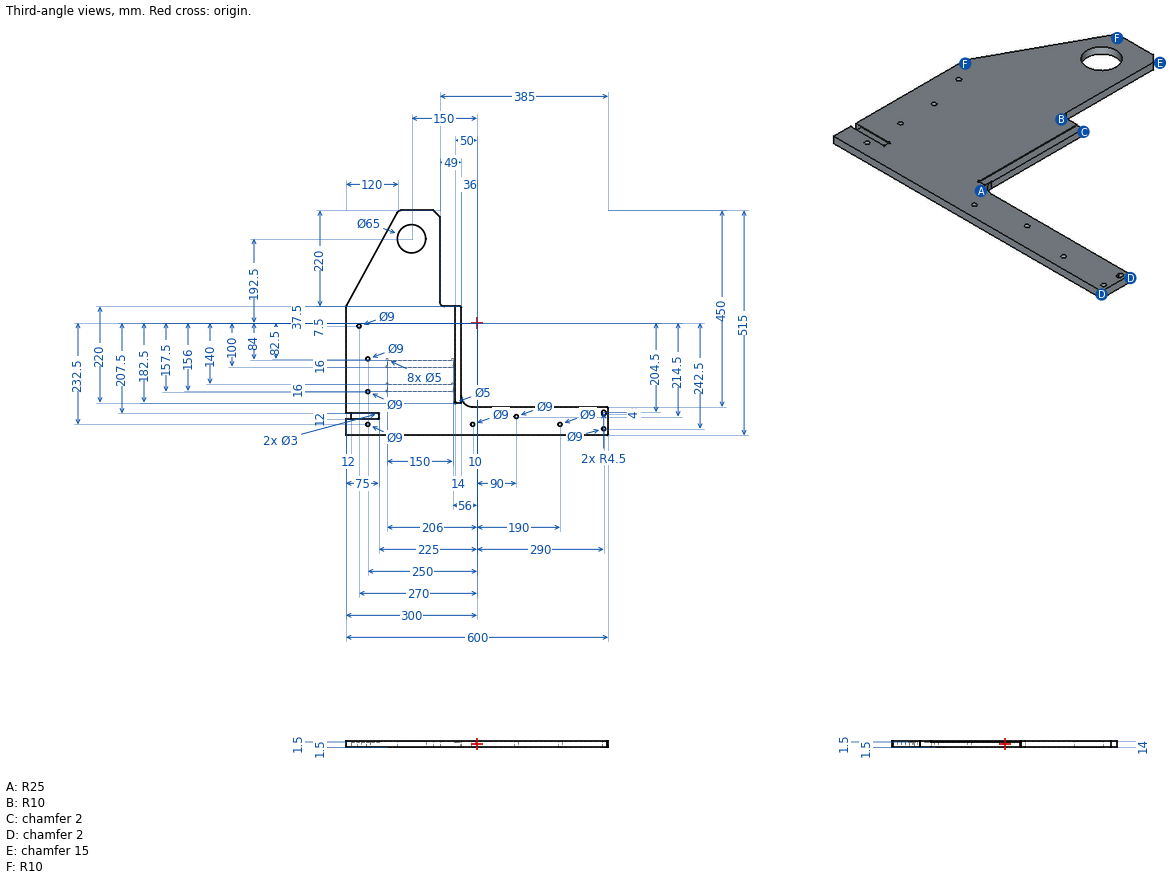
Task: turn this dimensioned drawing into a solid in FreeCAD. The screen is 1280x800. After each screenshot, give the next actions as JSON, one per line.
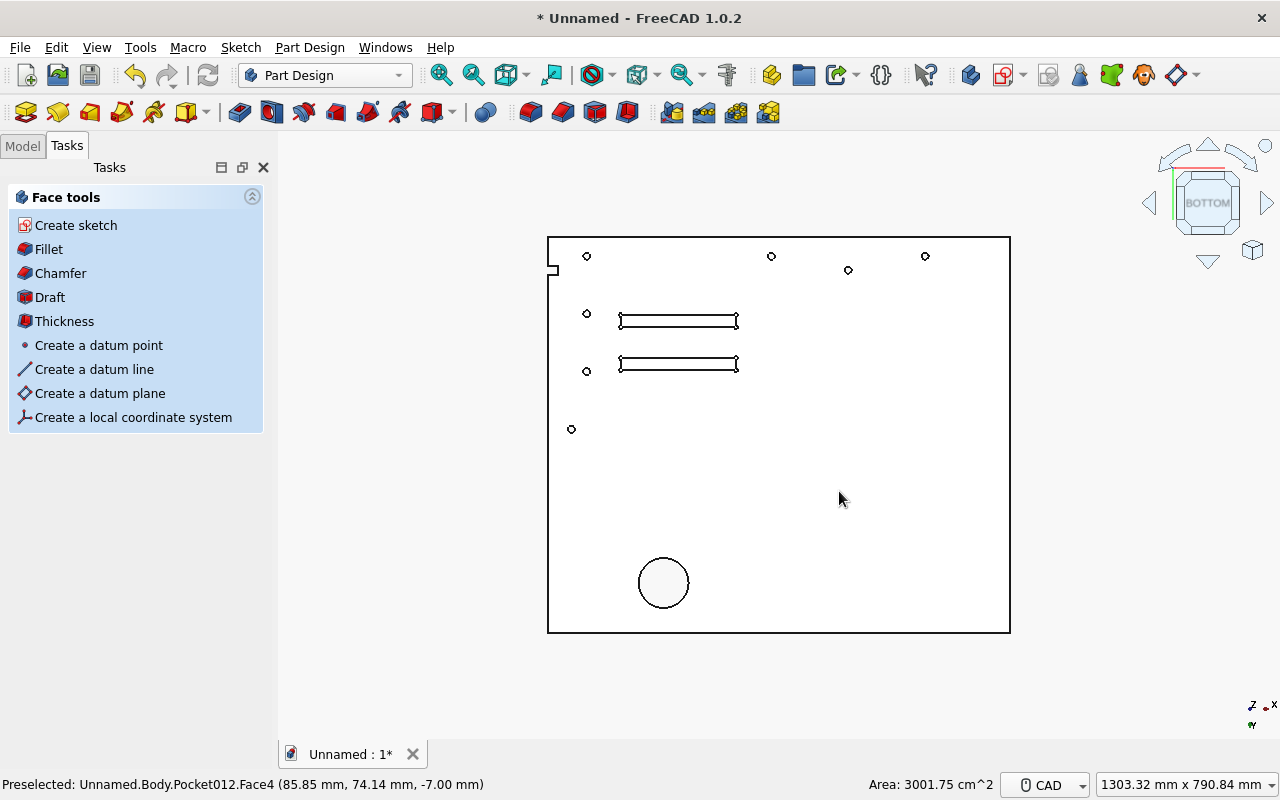
{"action": "left_click", "coordinate": [1004, 76]}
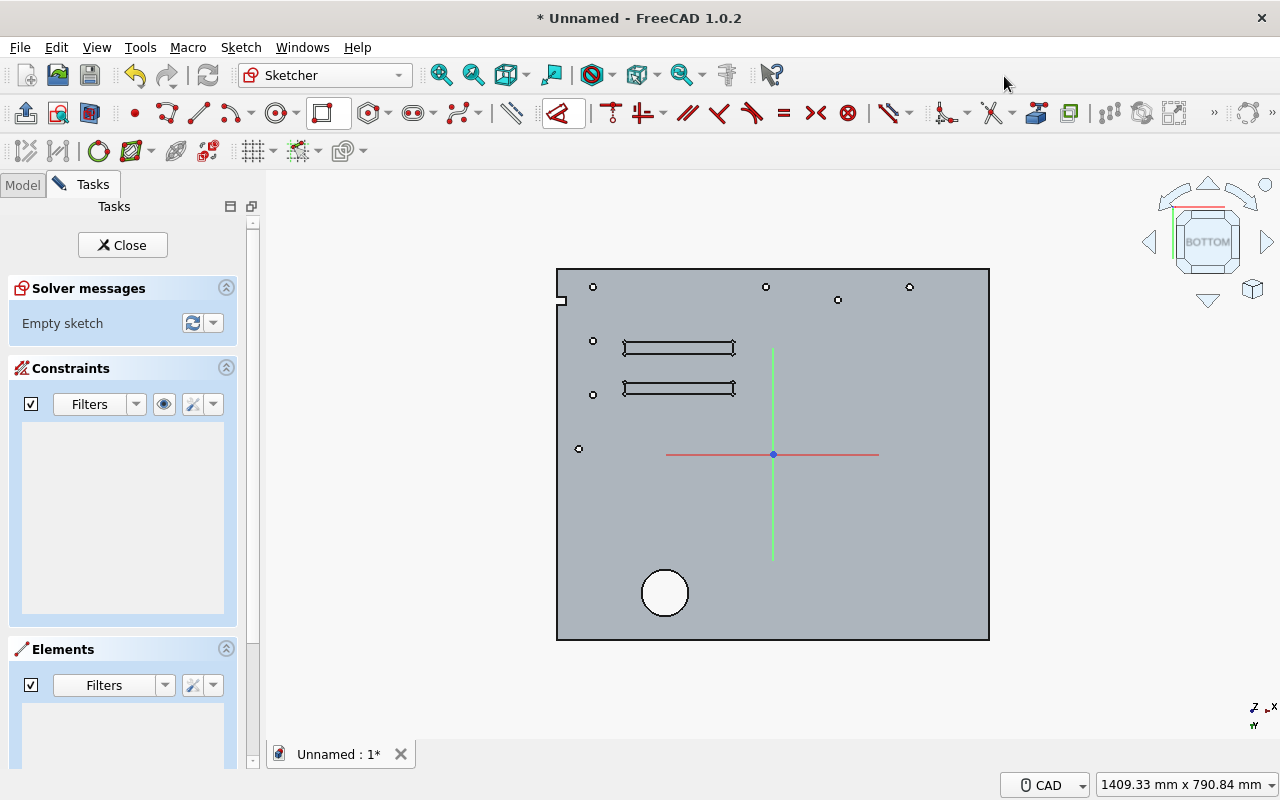
{"action": "scroll", "coordinate": [996, 271], "scroll_direction": "up", "scroll_amount": 15}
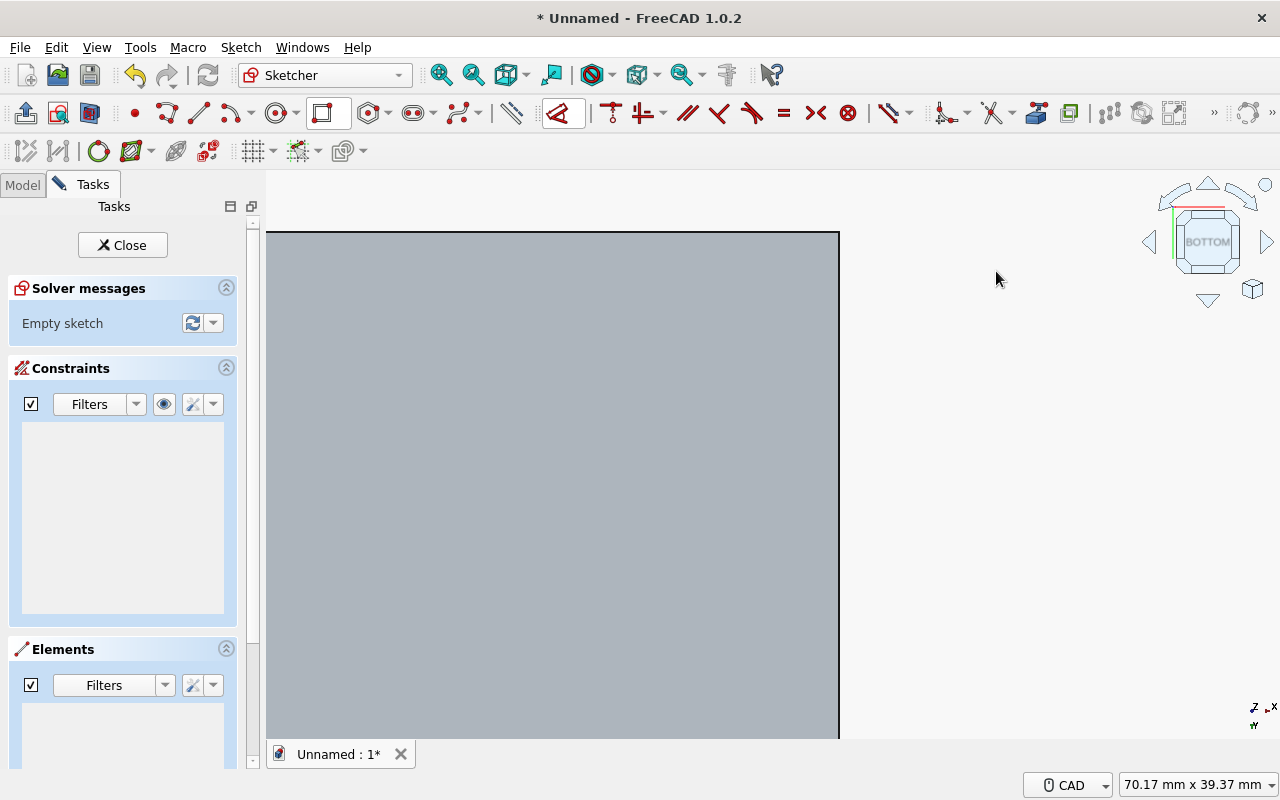
{"action": "scroll", "coordinate": [688, 446], "scroll_direction": "up", "scroll_amount": 5}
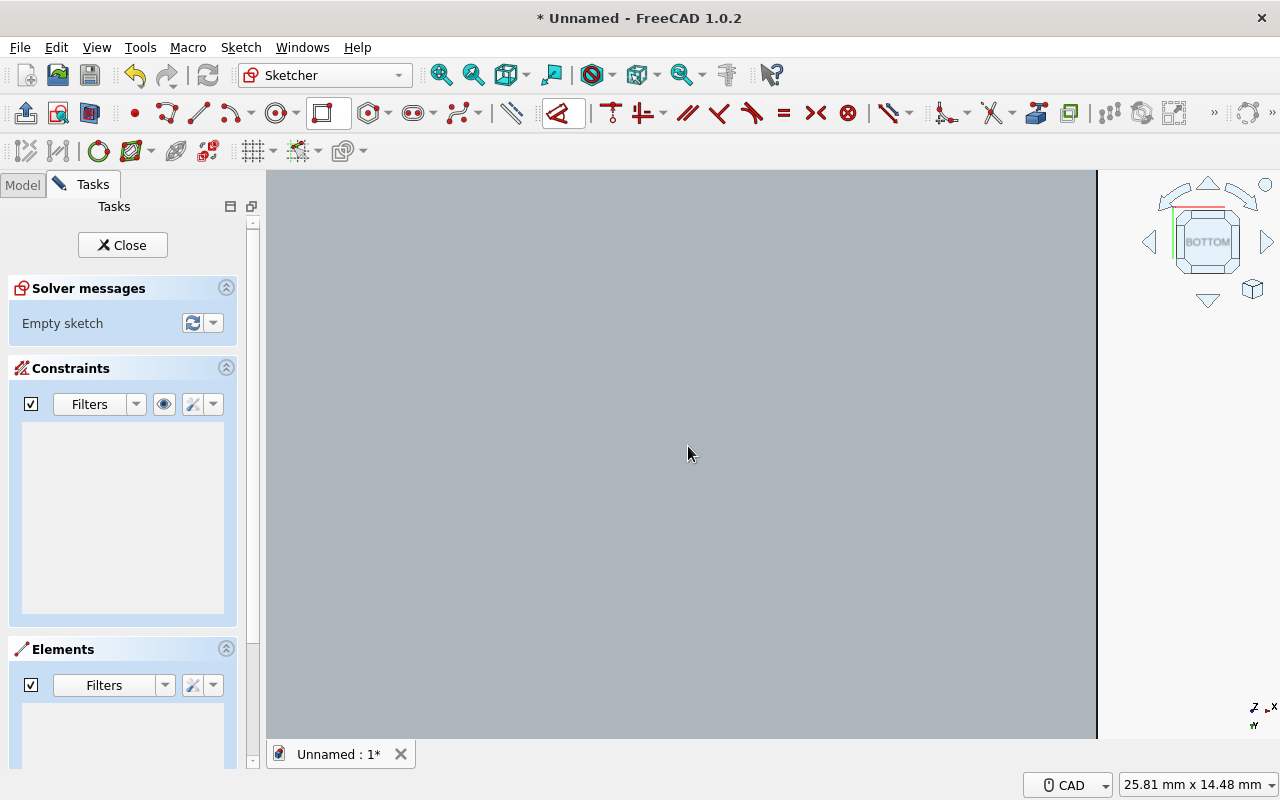
{"action": "left_click", "coordinate": [276, 114]}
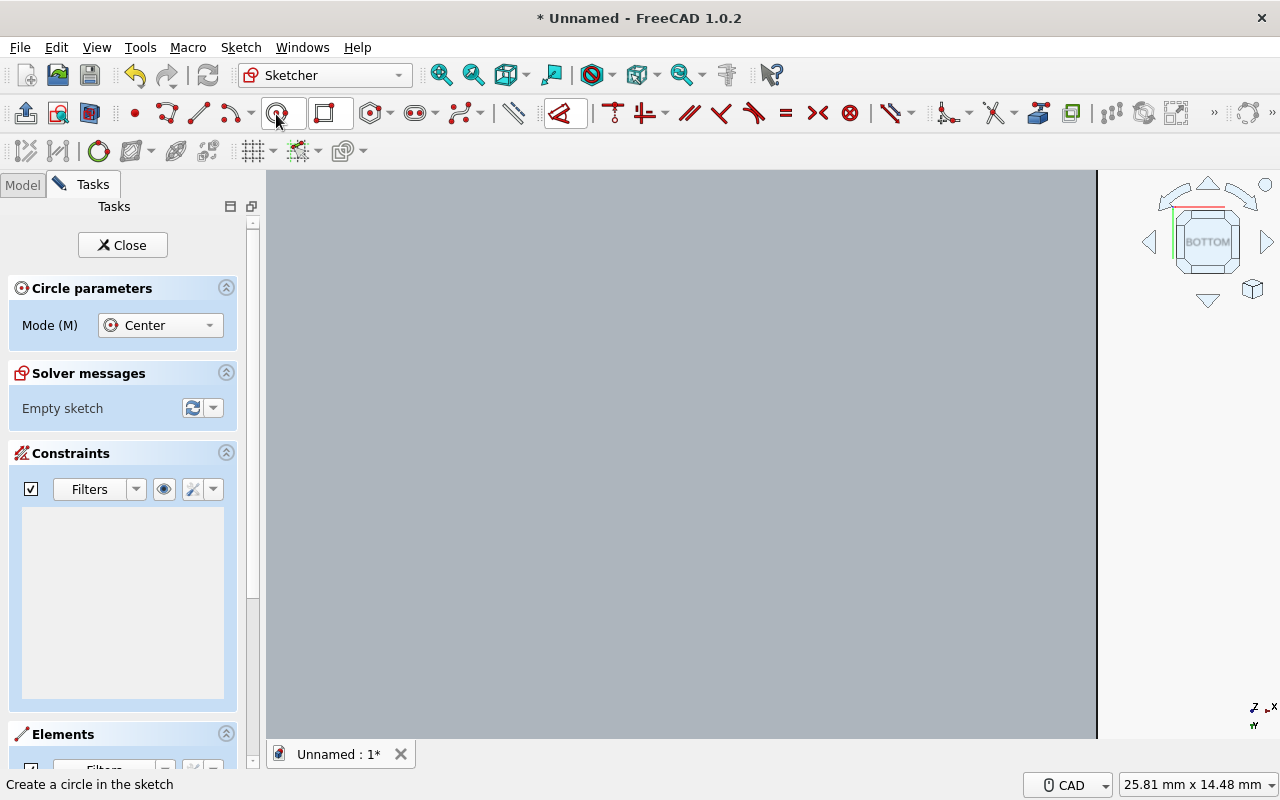
{"action": "left_click", "coordinate": [704, 453]}
{"action": "mouse_move", "coordinate": [829, 328]}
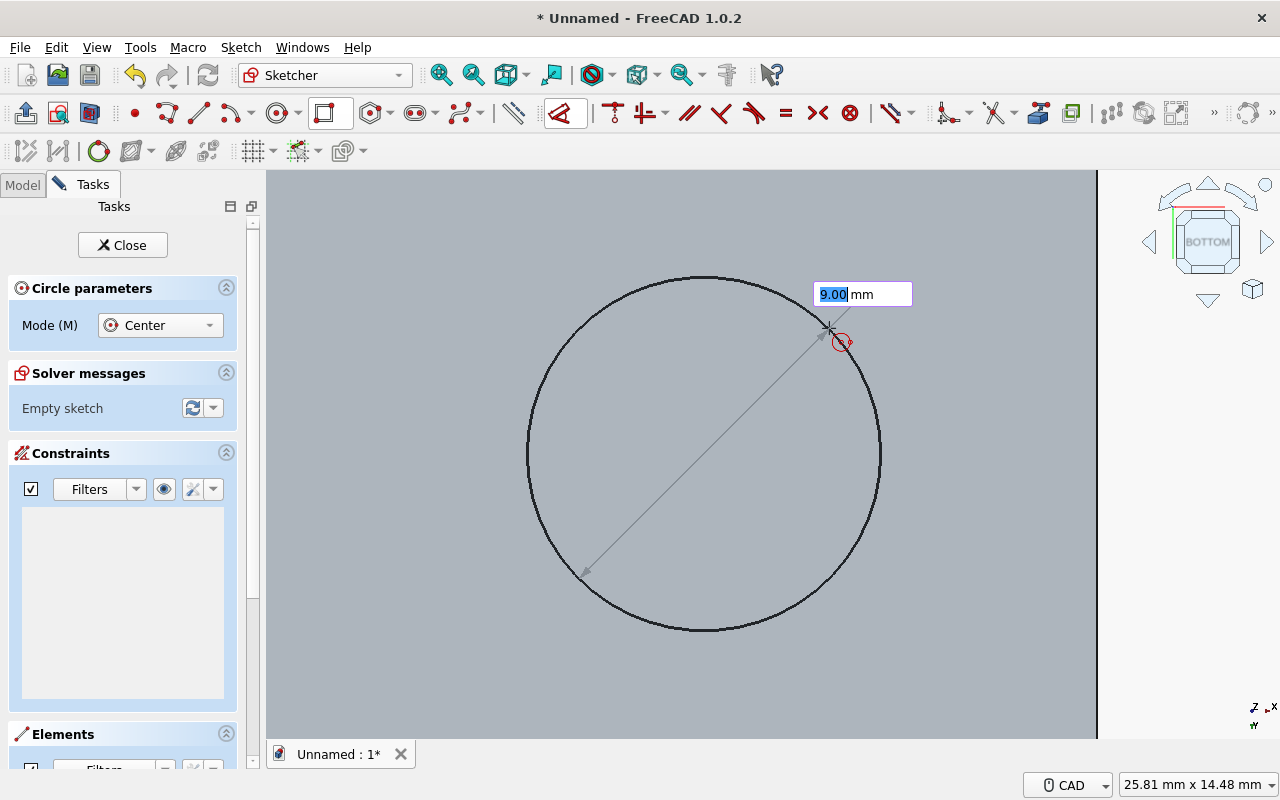
{"action": "type", "text": "9"}
{"action": "key", "text": "Return"}
{"action": "key", "text": "Escape"}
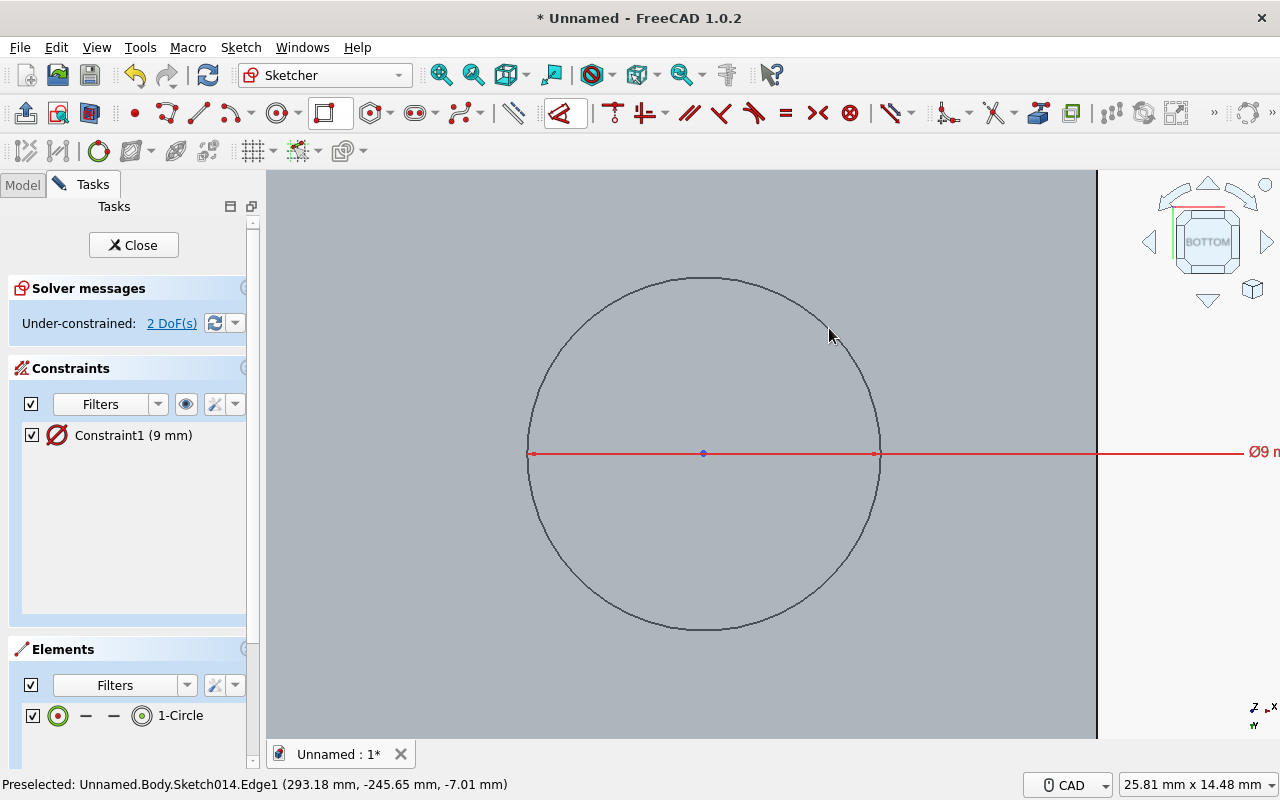
{"action": "left_click", "coordinate": [704, 454]}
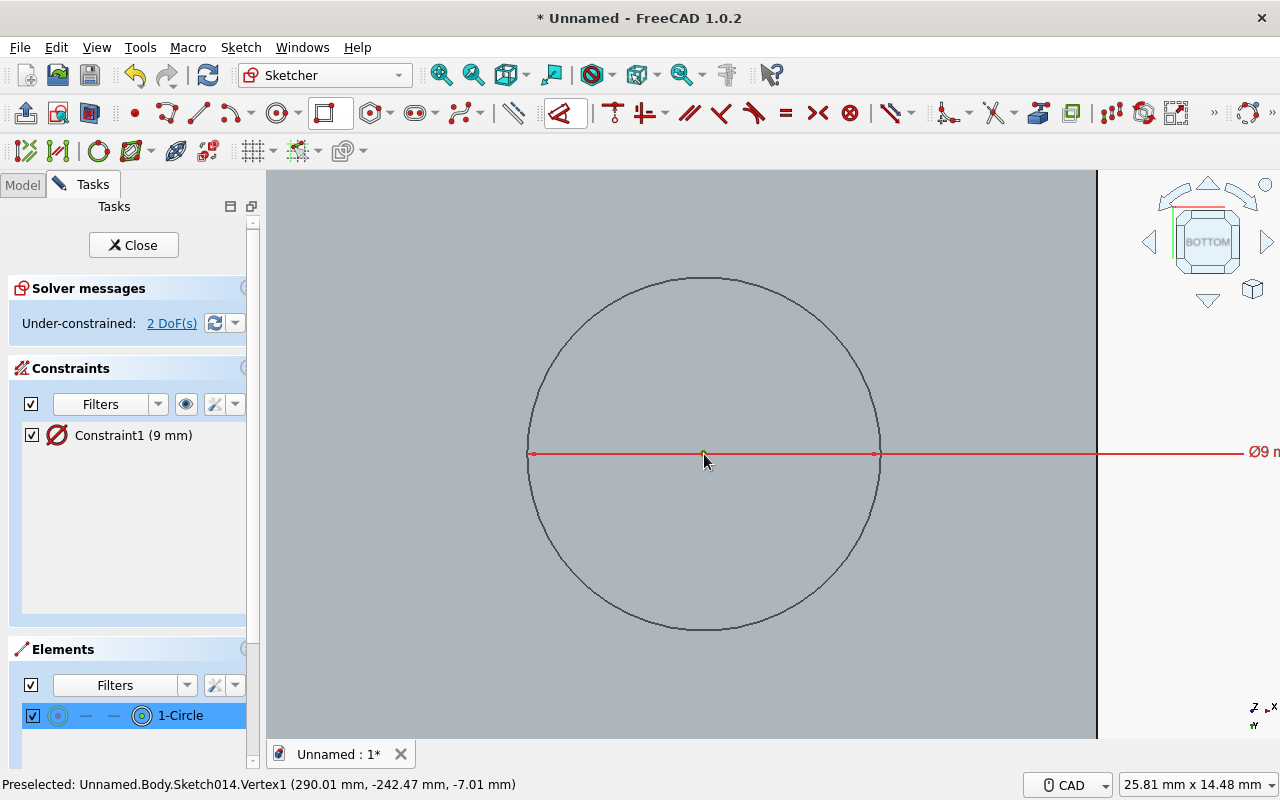
{"action": "left_click", "coordinate": [582, 114]}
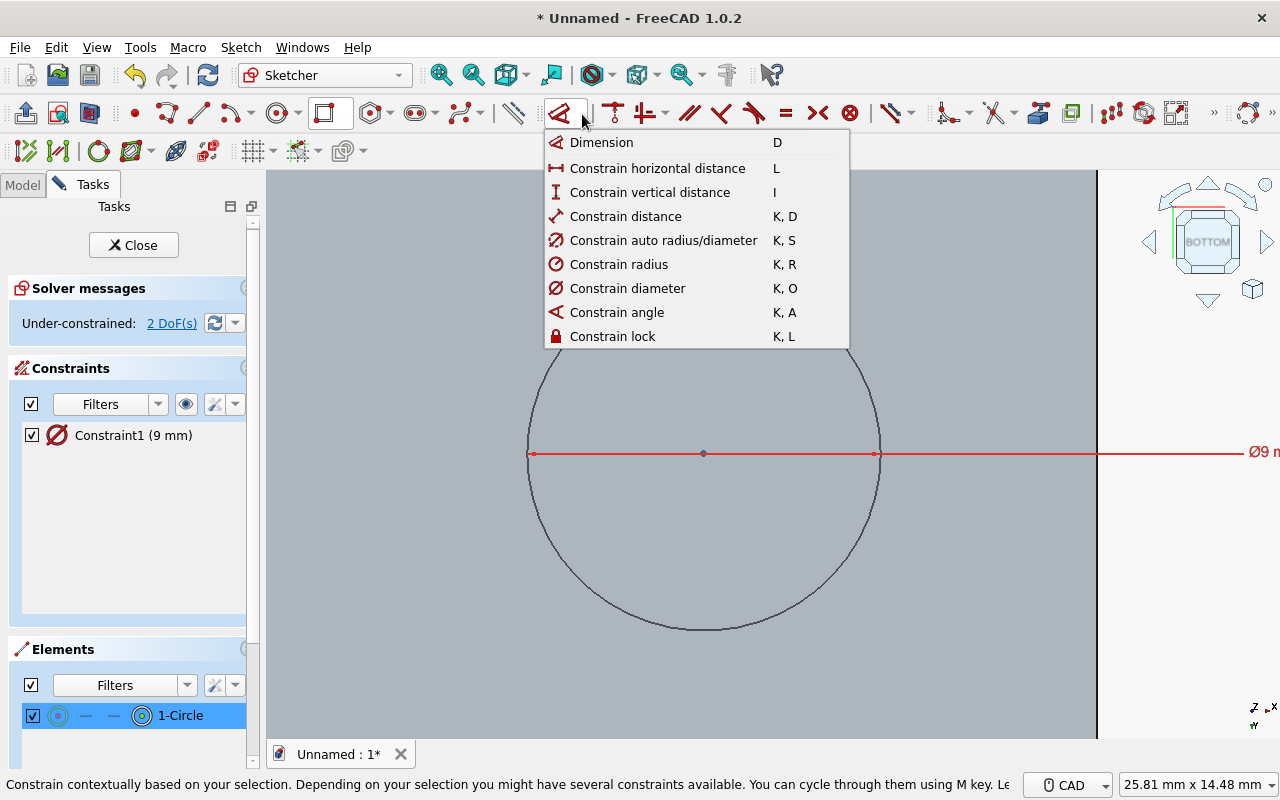
{"action": "left_click", "coordinate": [697, 168]}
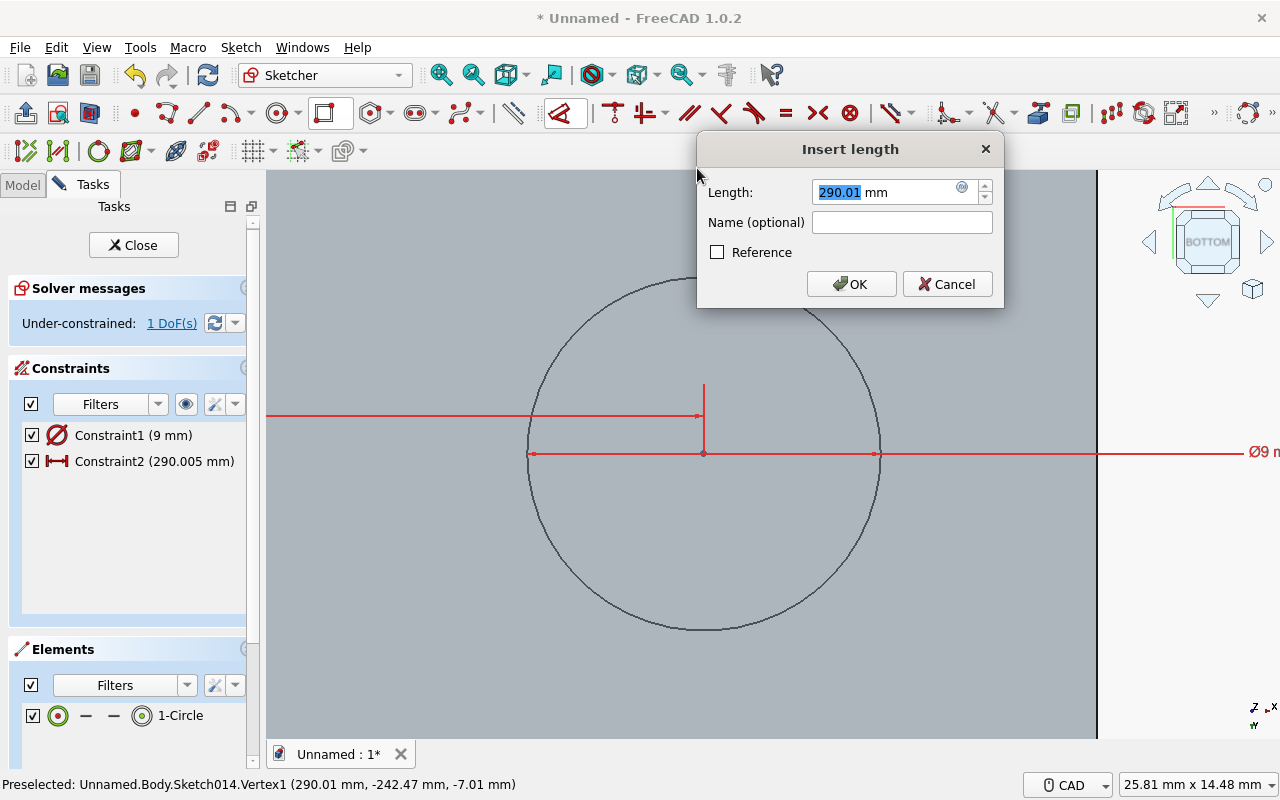
{"action": "type", "text": "290"}
{"action": "key", "text": "Return"}